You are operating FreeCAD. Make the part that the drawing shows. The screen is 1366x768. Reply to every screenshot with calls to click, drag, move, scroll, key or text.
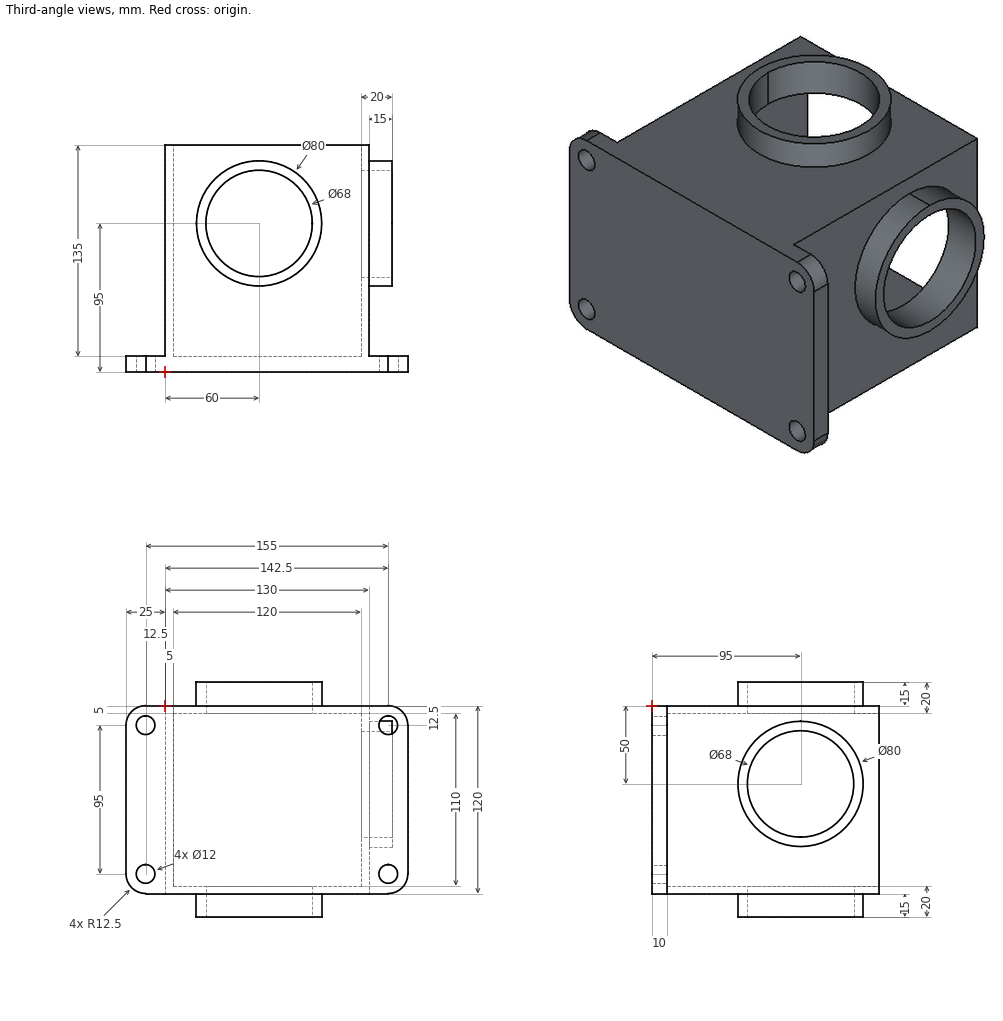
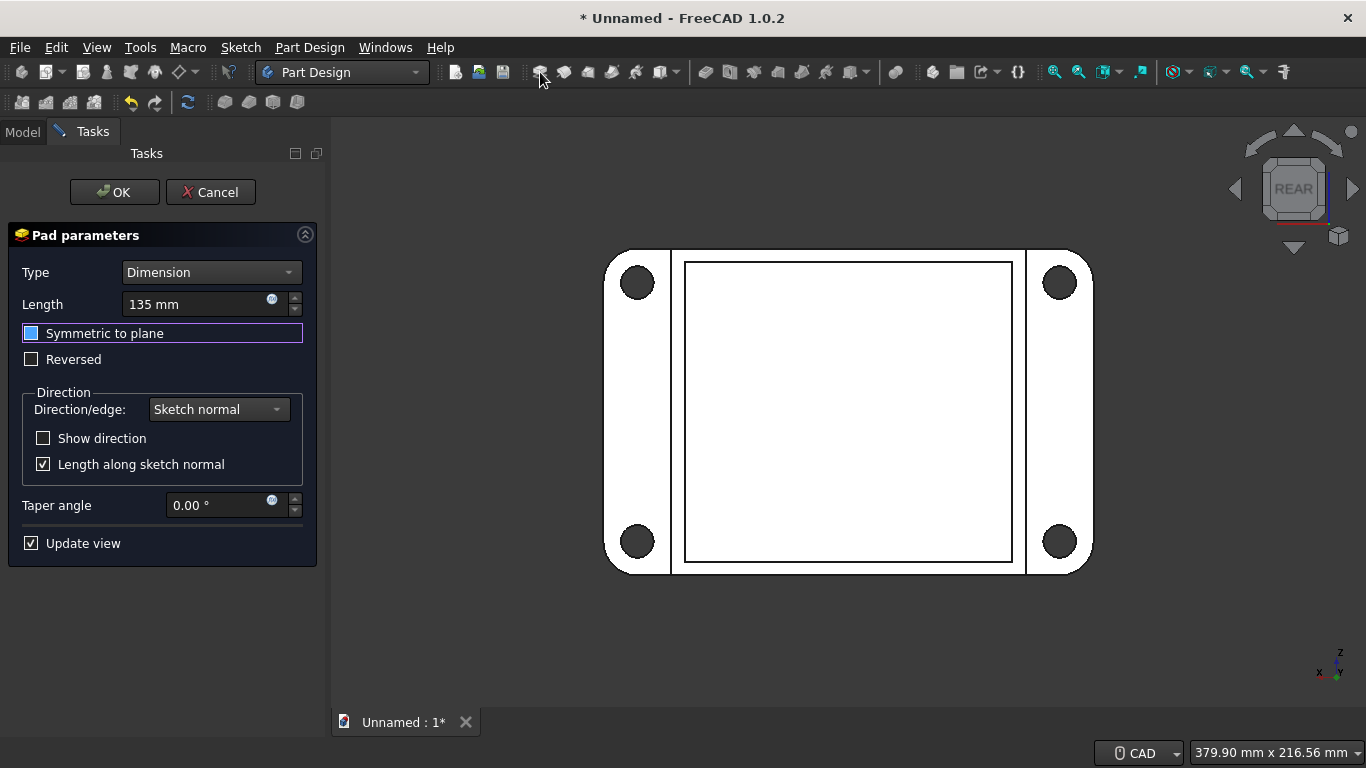
click(115, 192)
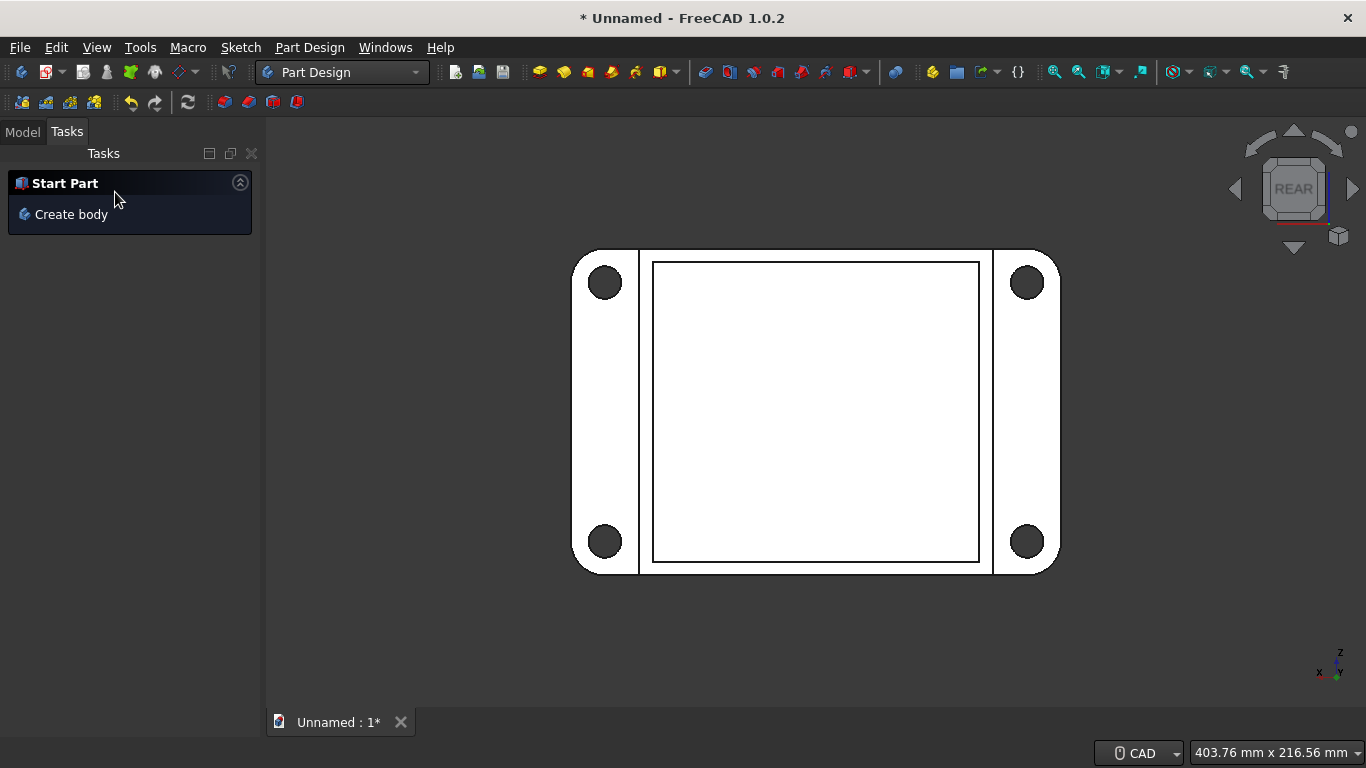
key(0)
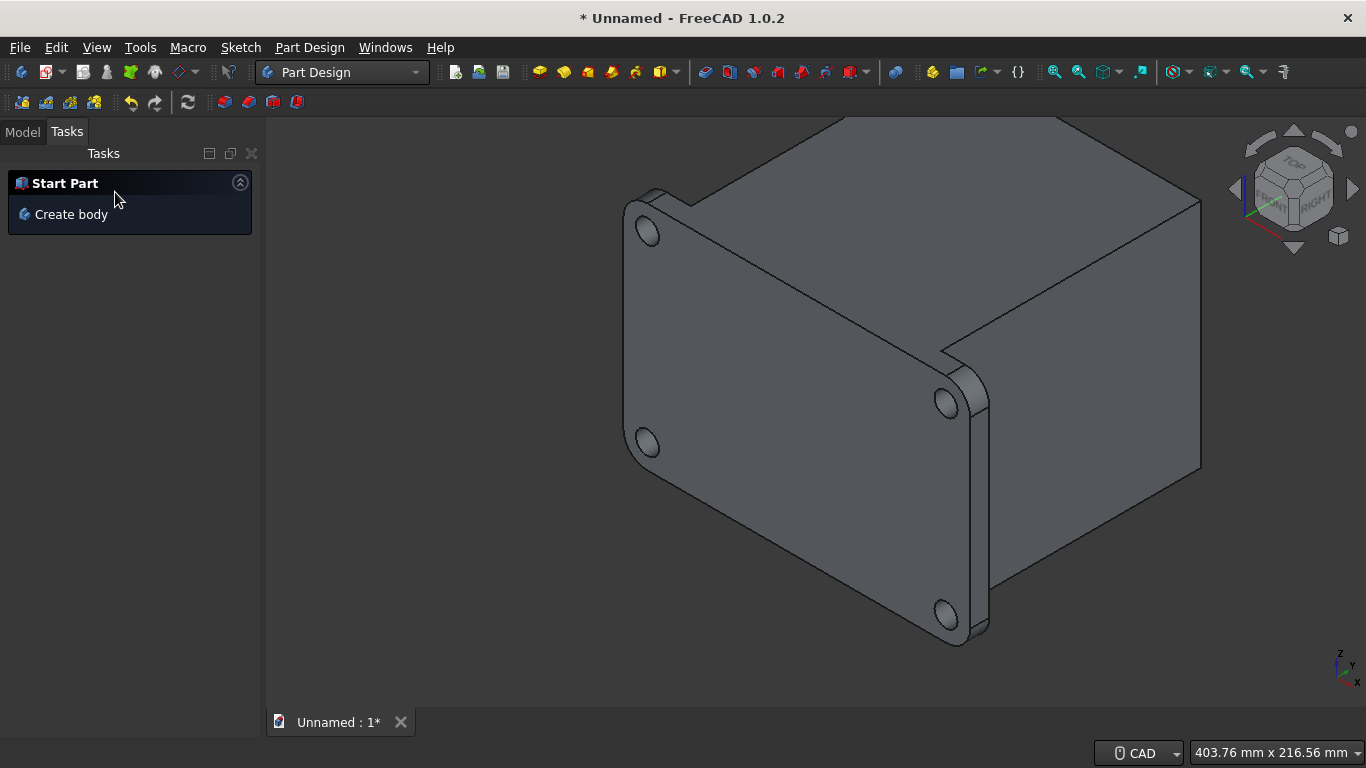
click(1056, 72)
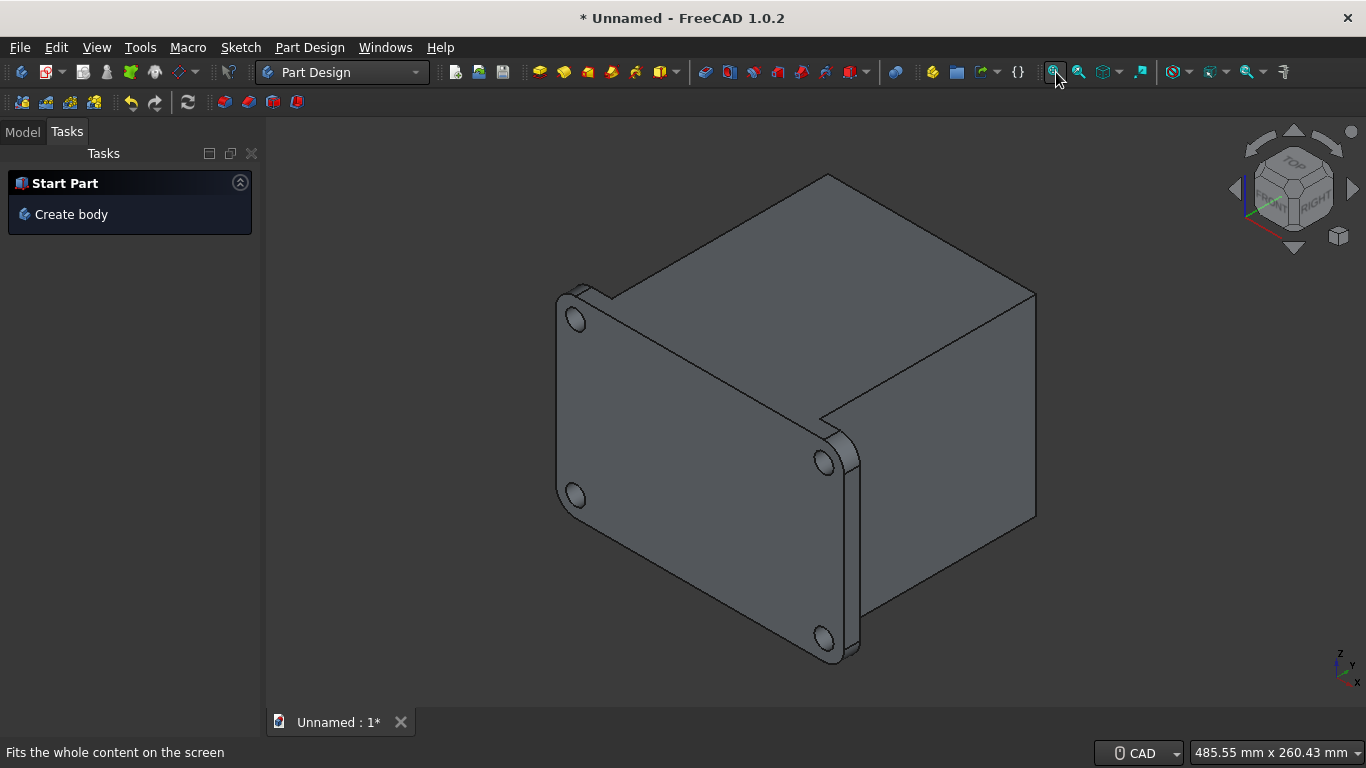
click(816, 300)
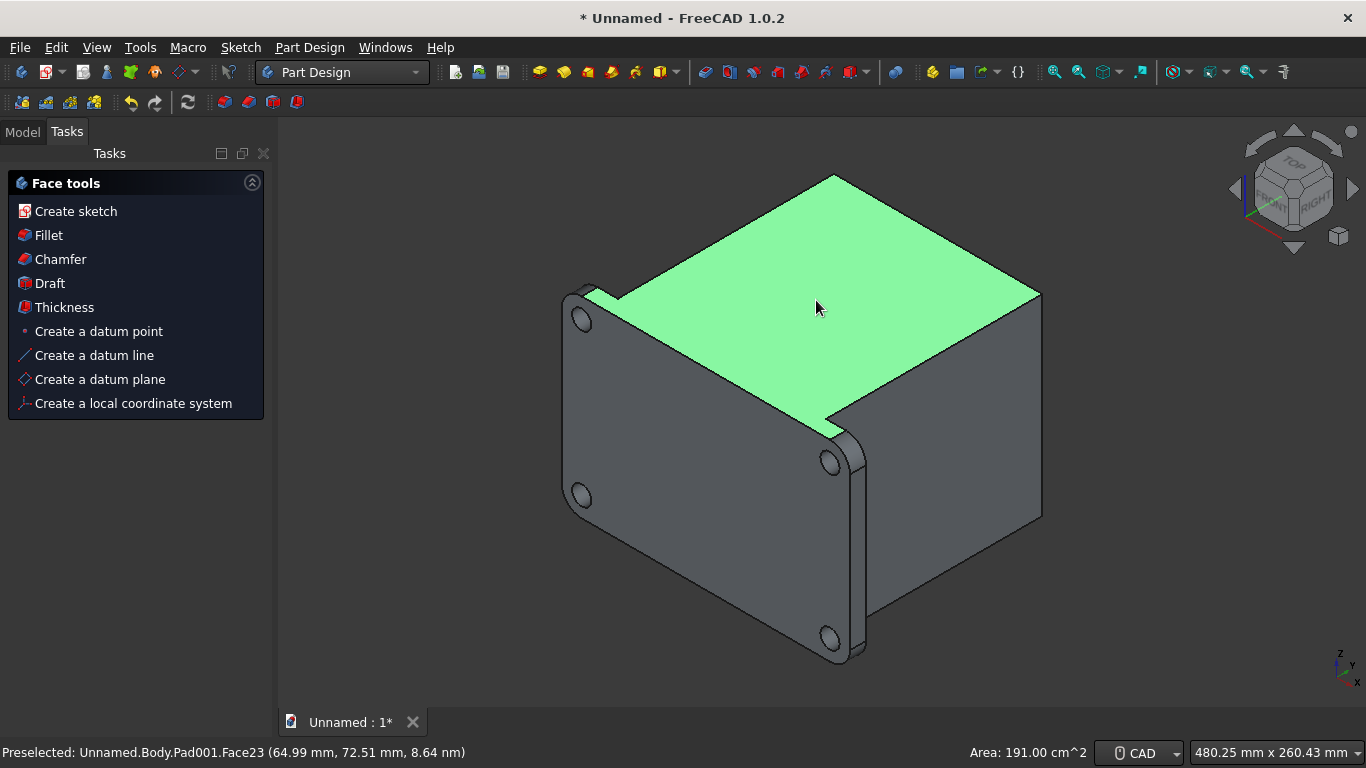
click(46, 72)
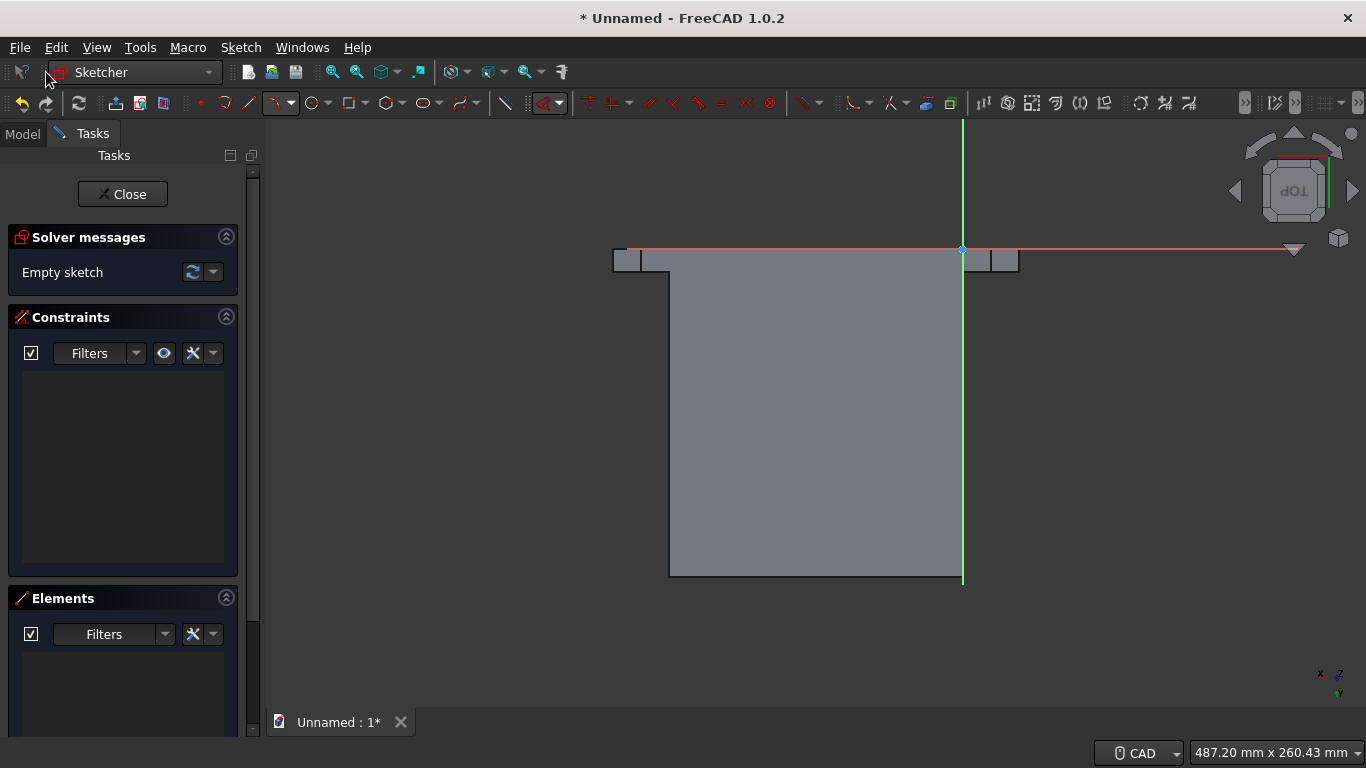
click(312, 104)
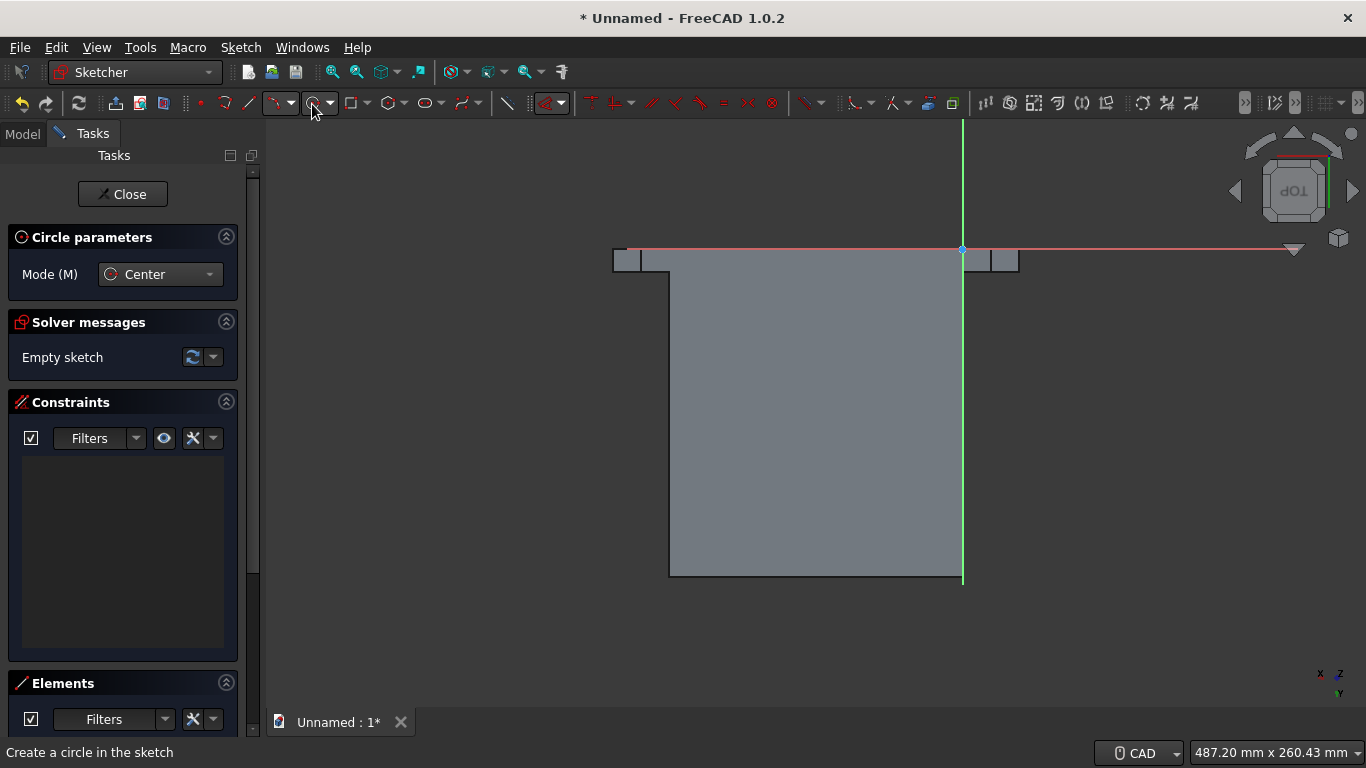
click(827, 464)
move(891, 400)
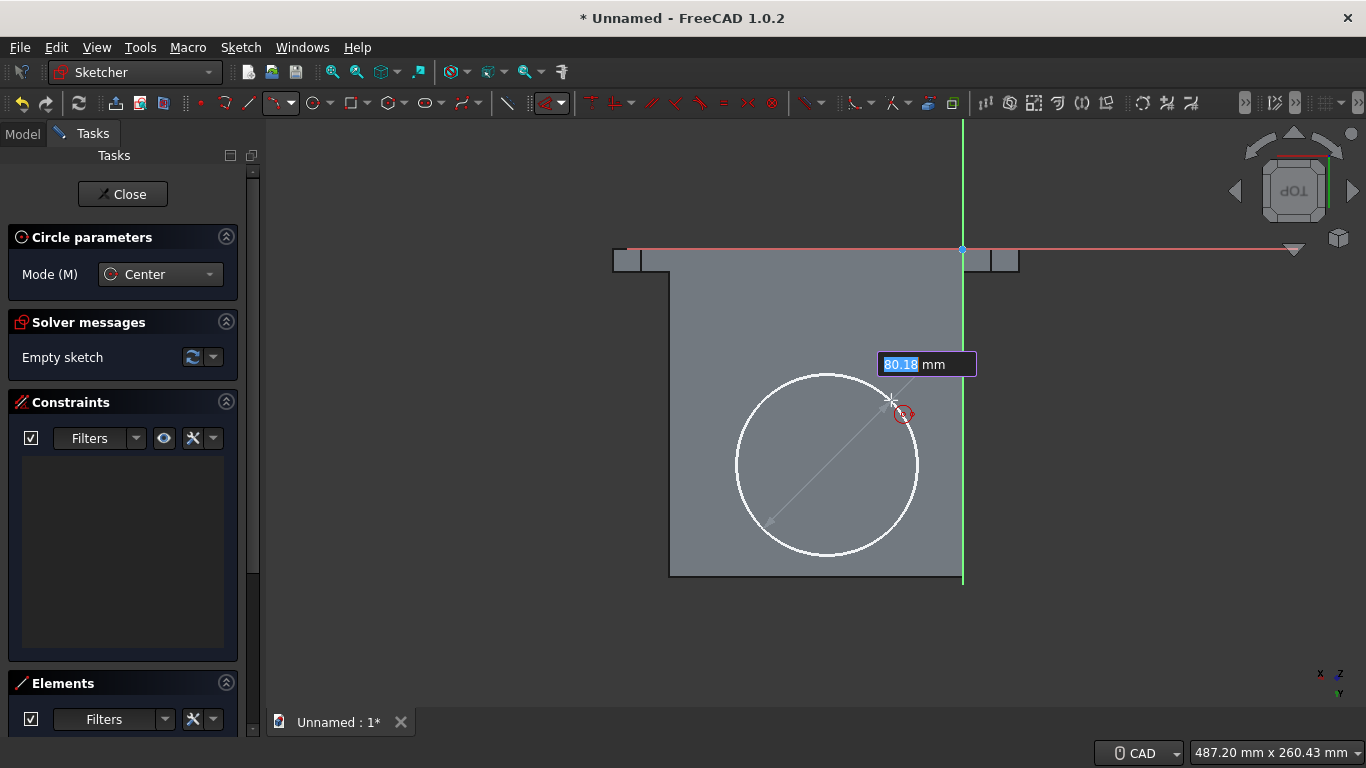
text(80)
key(Return)
key(Escape)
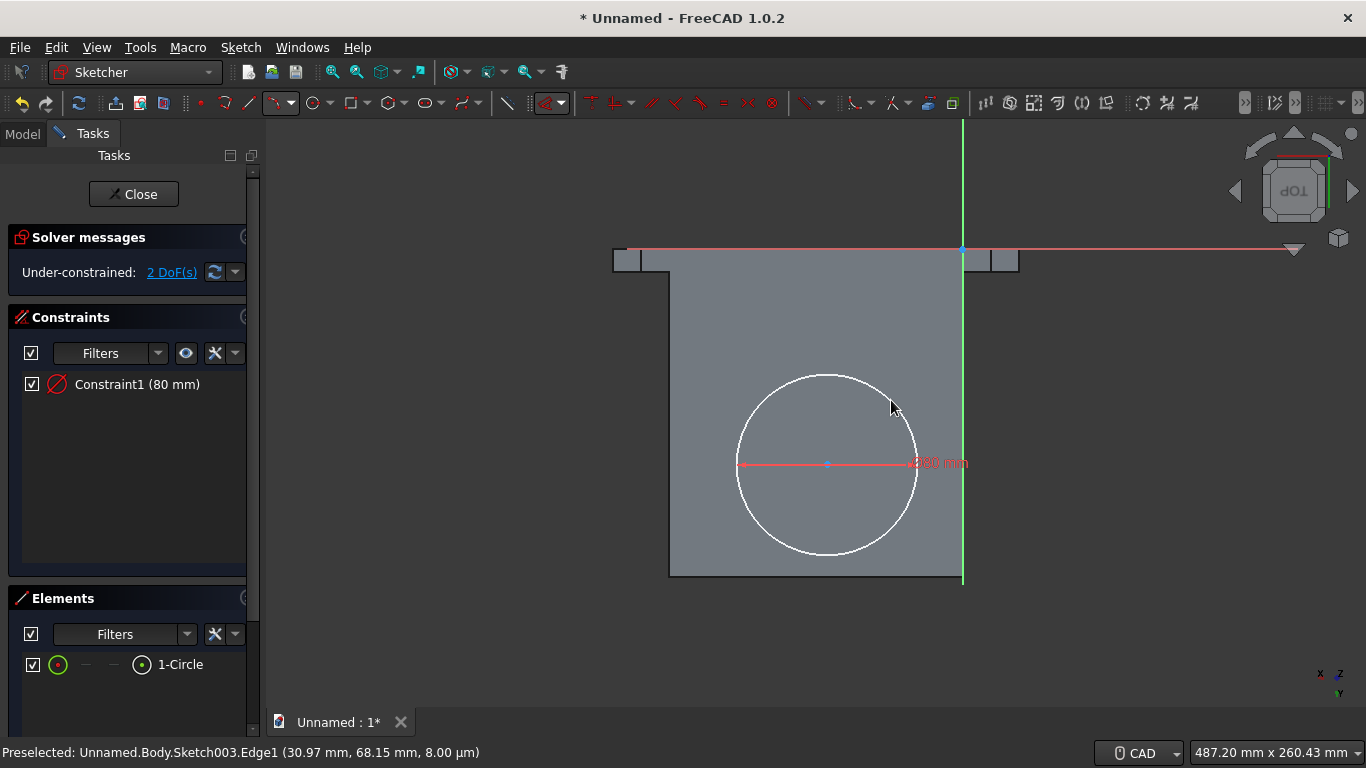
click(827, 465)